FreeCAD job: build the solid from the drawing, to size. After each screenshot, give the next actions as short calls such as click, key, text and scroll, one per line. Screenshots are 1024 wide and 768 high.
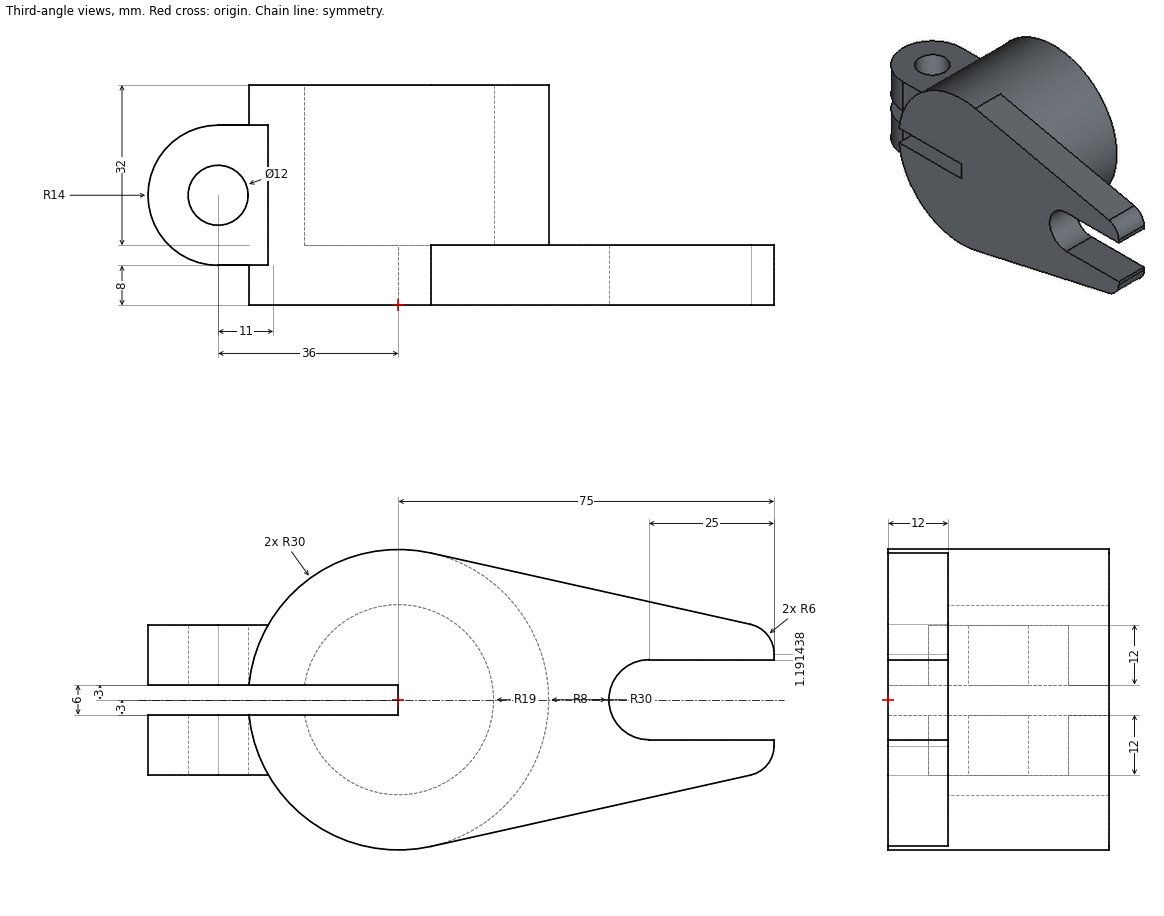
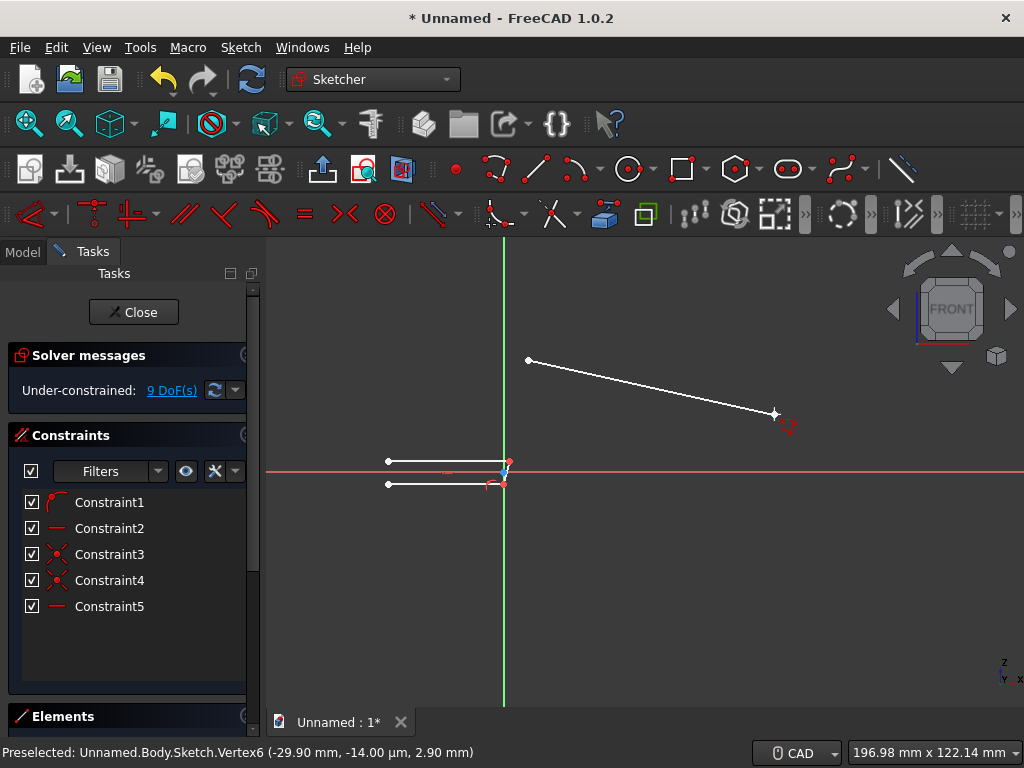
click(792, 437)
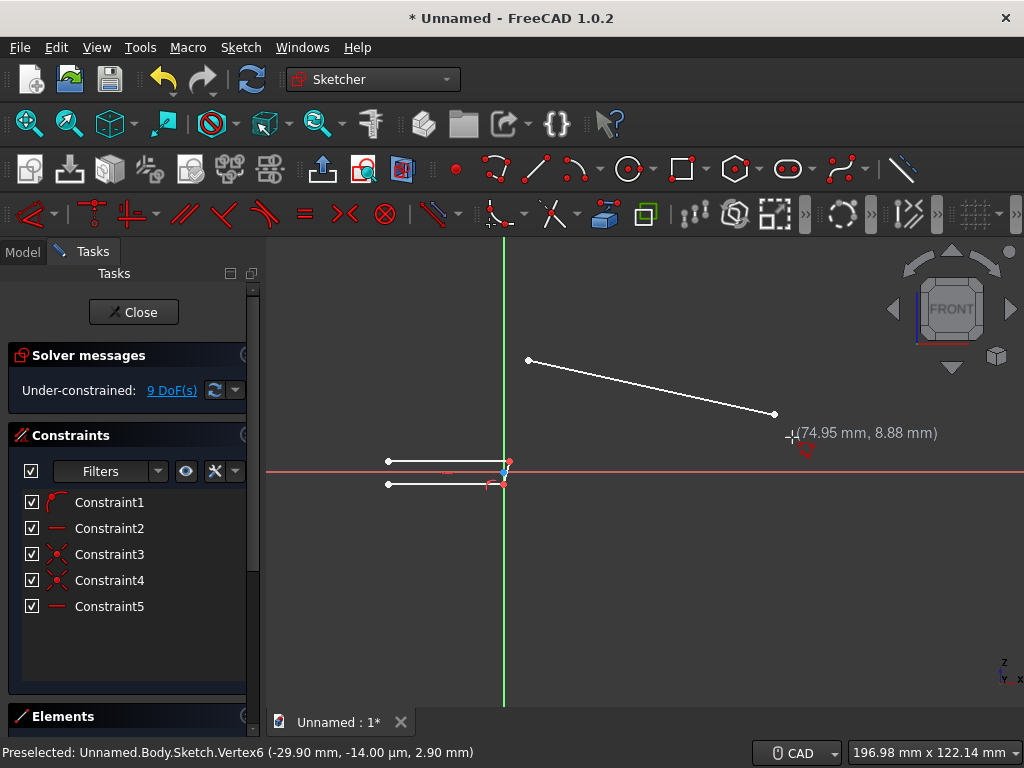
scroll(792, 441, up, 7)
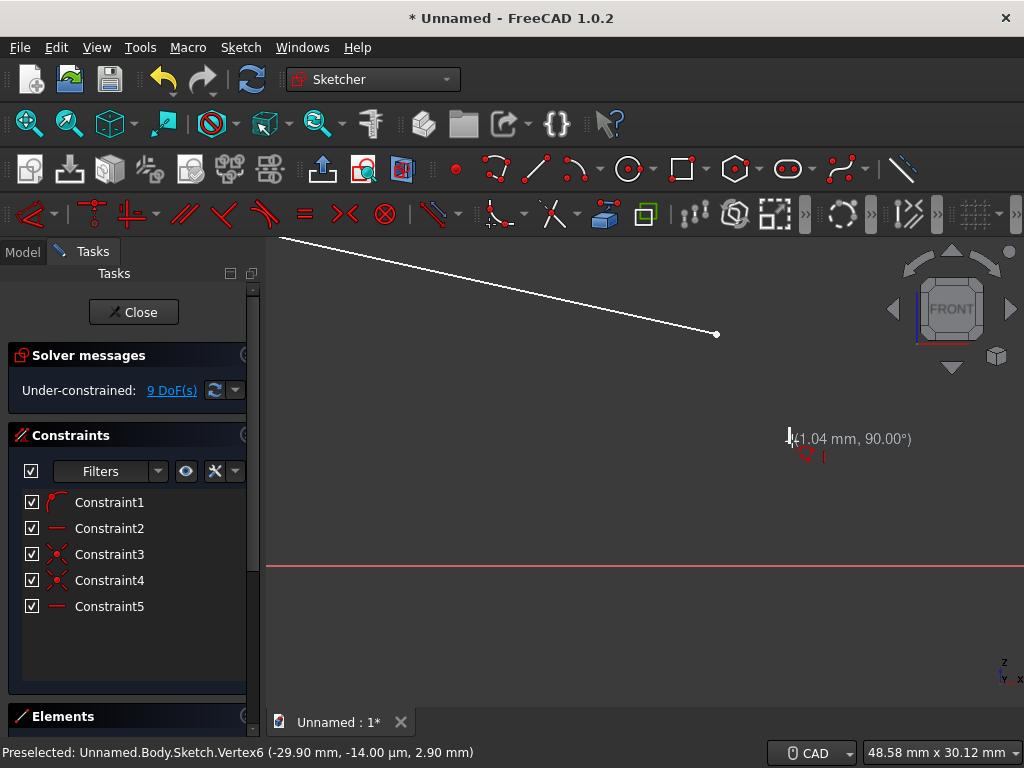
click(790, 441)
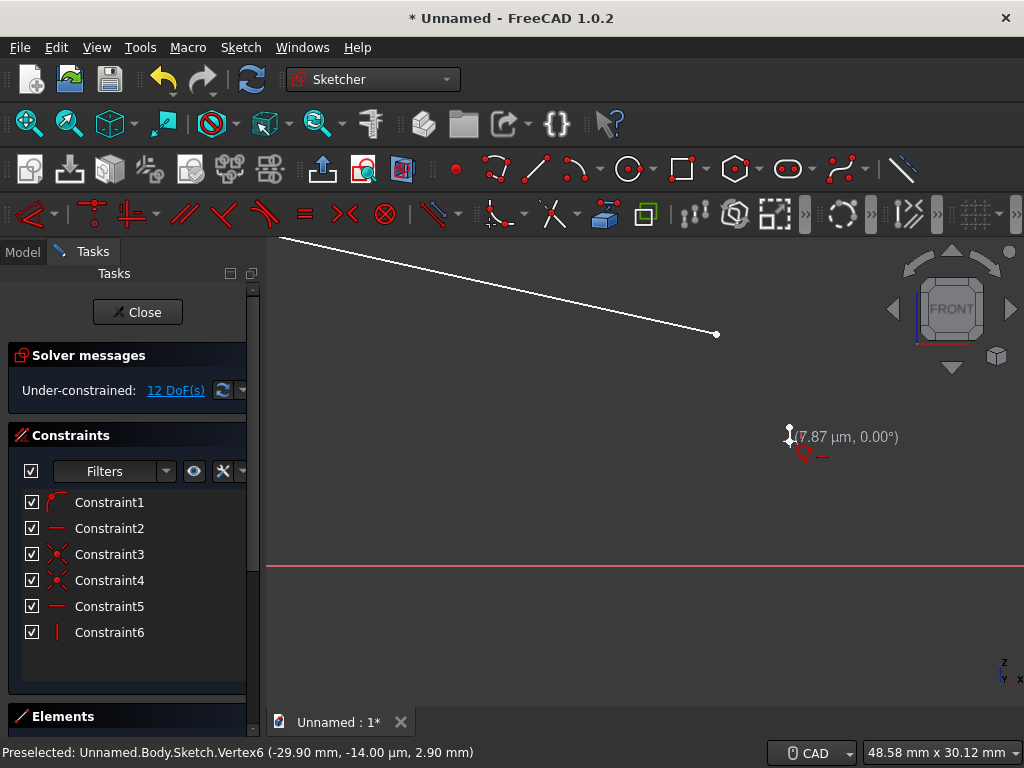
scroll(774, 441, down, 7)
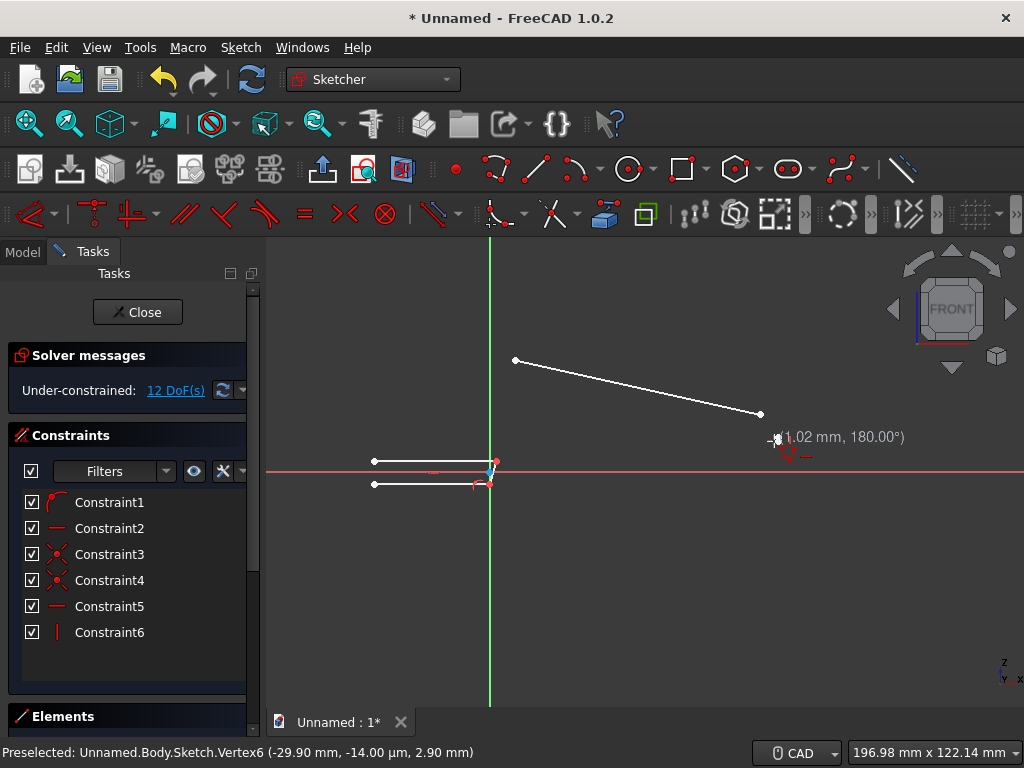
click(682, 441)
right_click(682, 441)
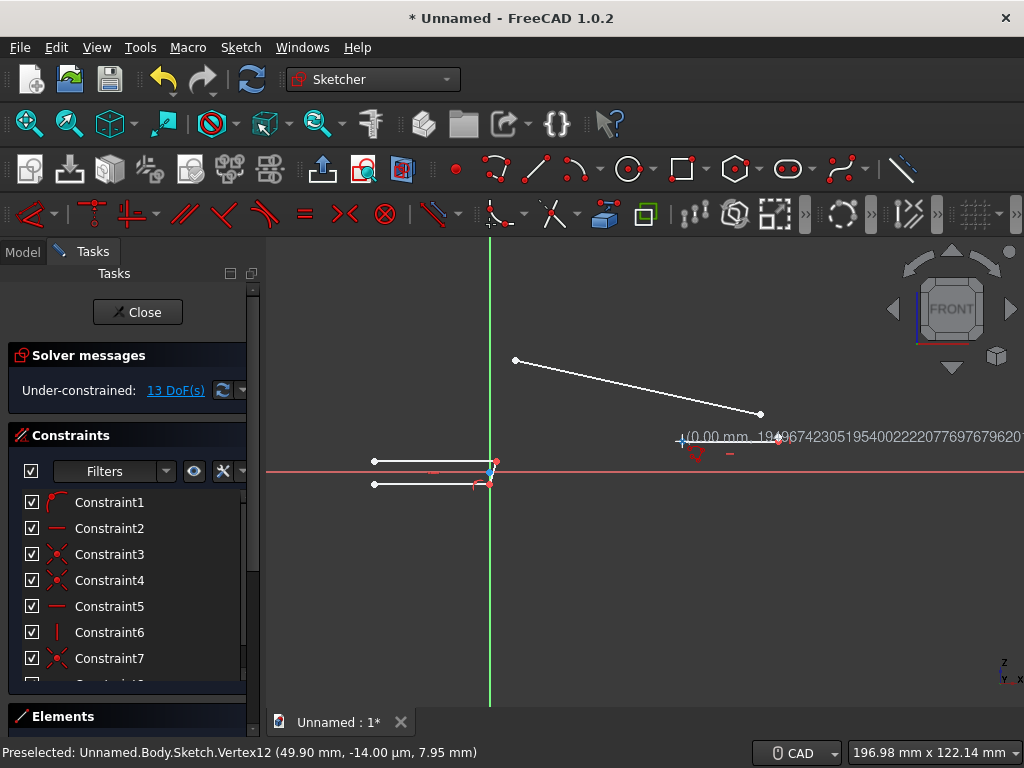
click(682, 503)
click(779, 503)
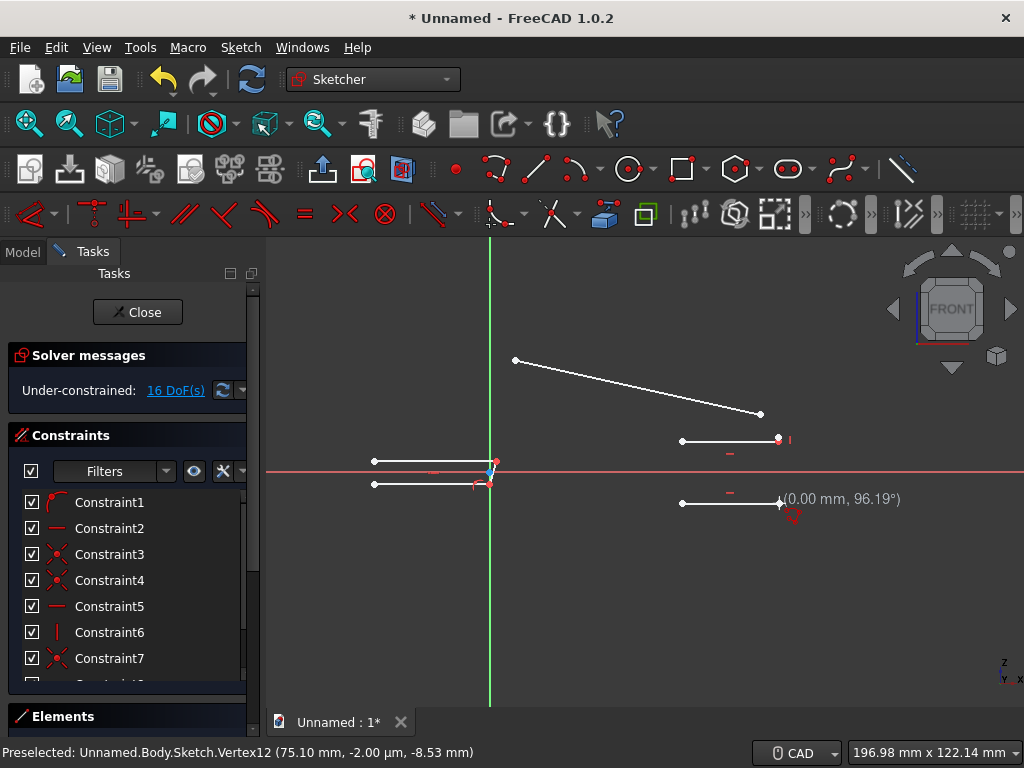
scroll(779, 508, up, 7)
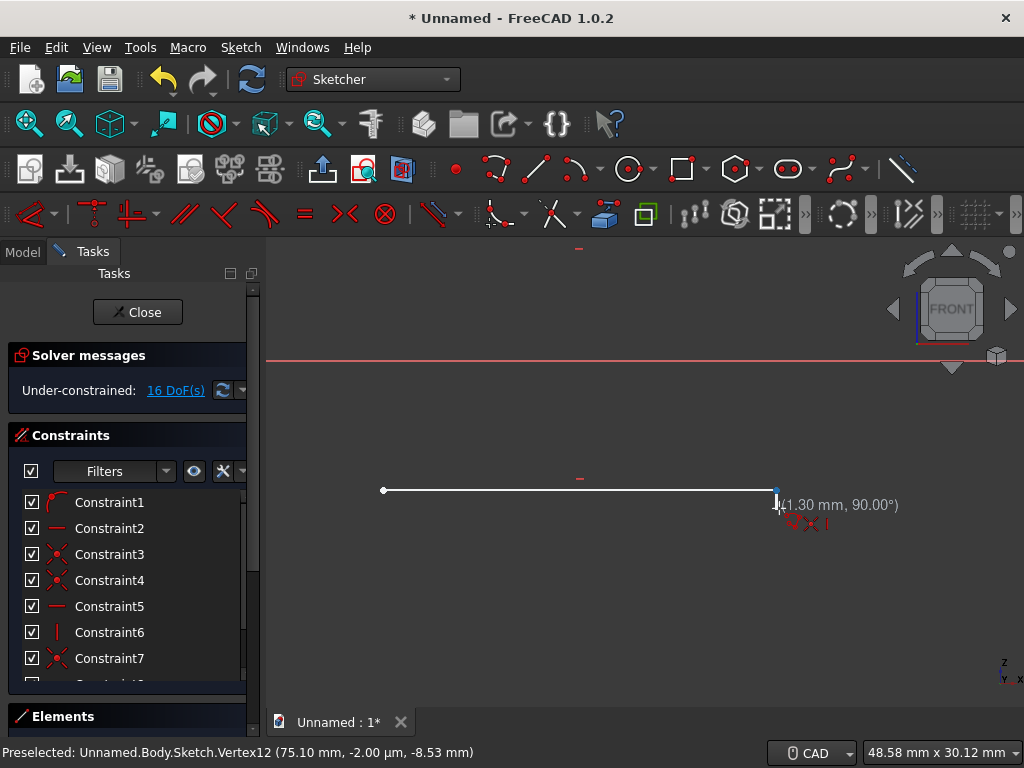
click(777, 504)
right_click(777, 504)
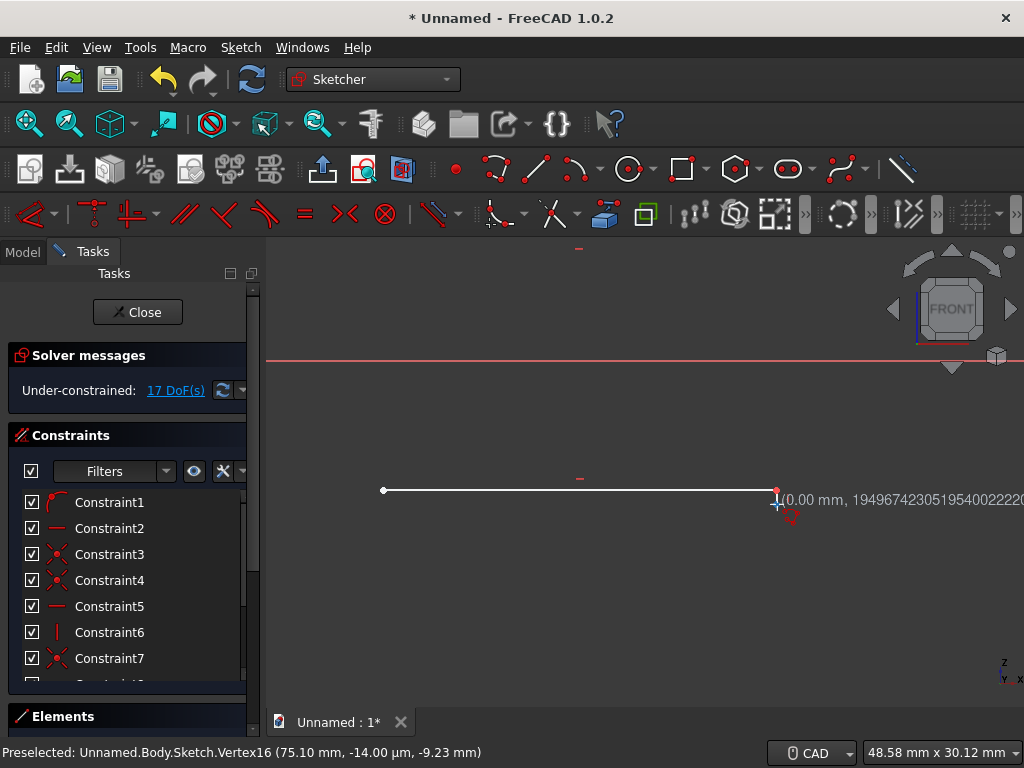
key(g)
key(l)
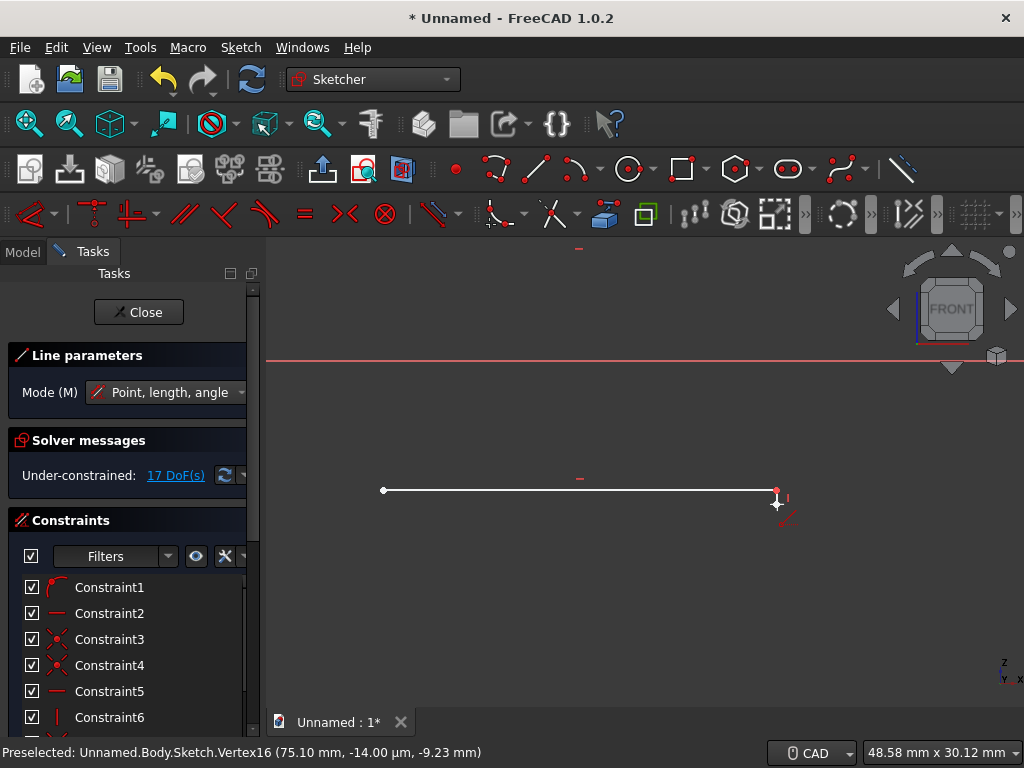
scroll(779, 508, down, 7)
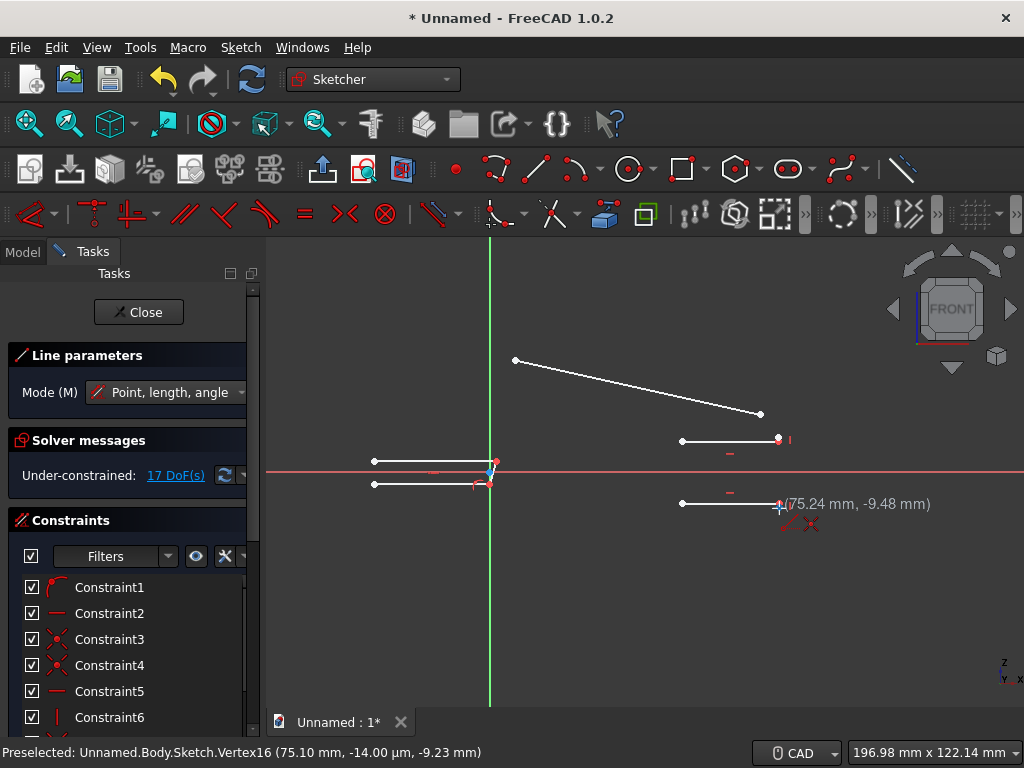
click(761, 530)
click(515, 585)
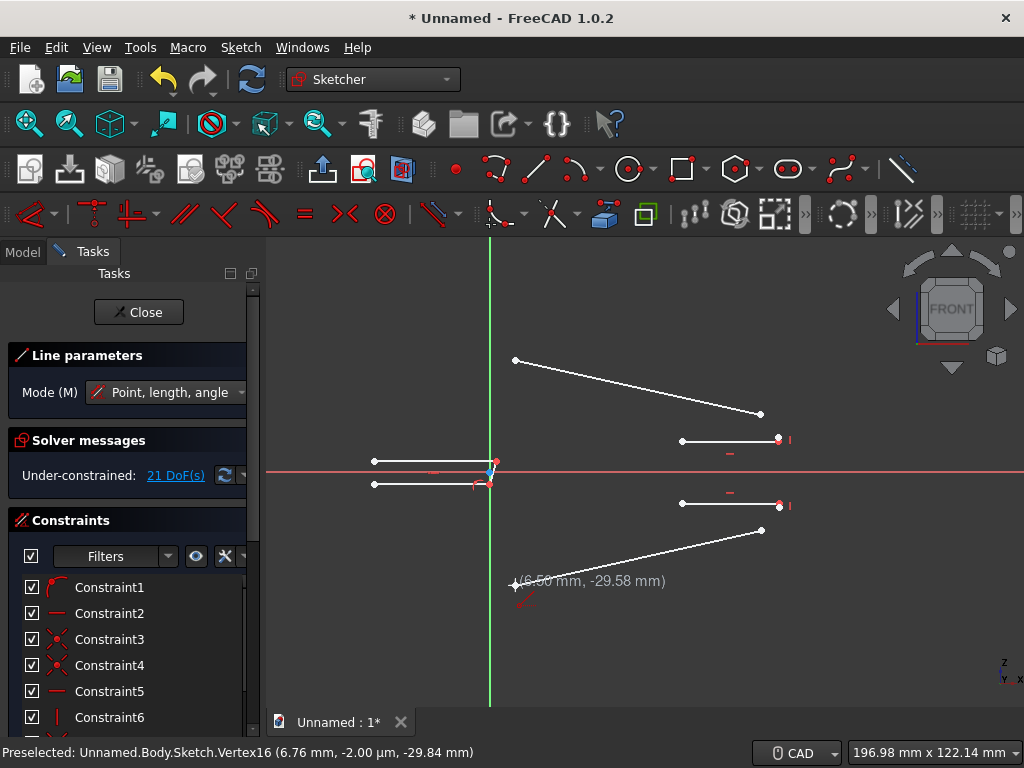
key(g)
key(3)
key(a)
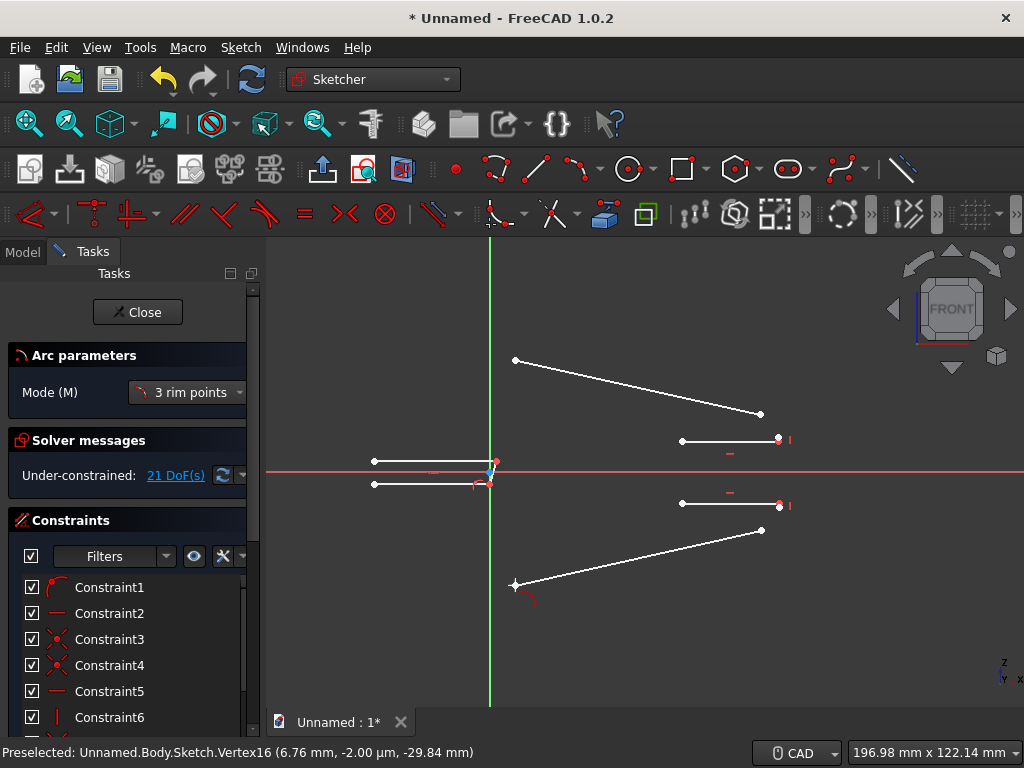
scroll(375, 461, up, 2)